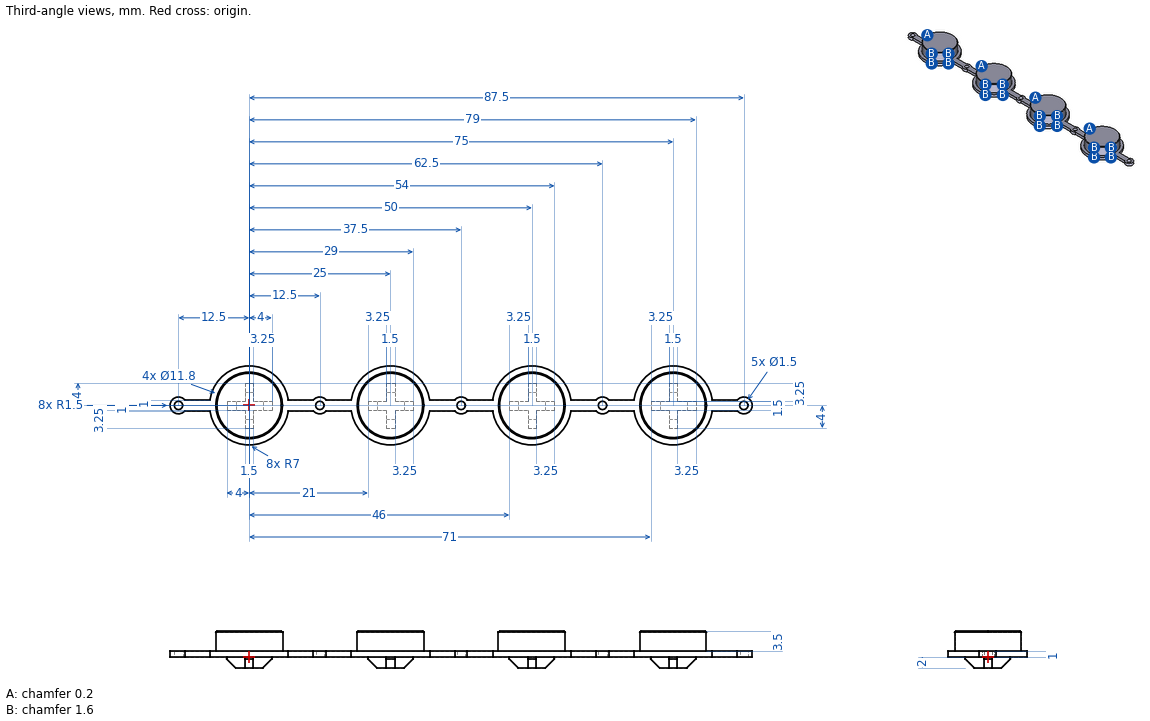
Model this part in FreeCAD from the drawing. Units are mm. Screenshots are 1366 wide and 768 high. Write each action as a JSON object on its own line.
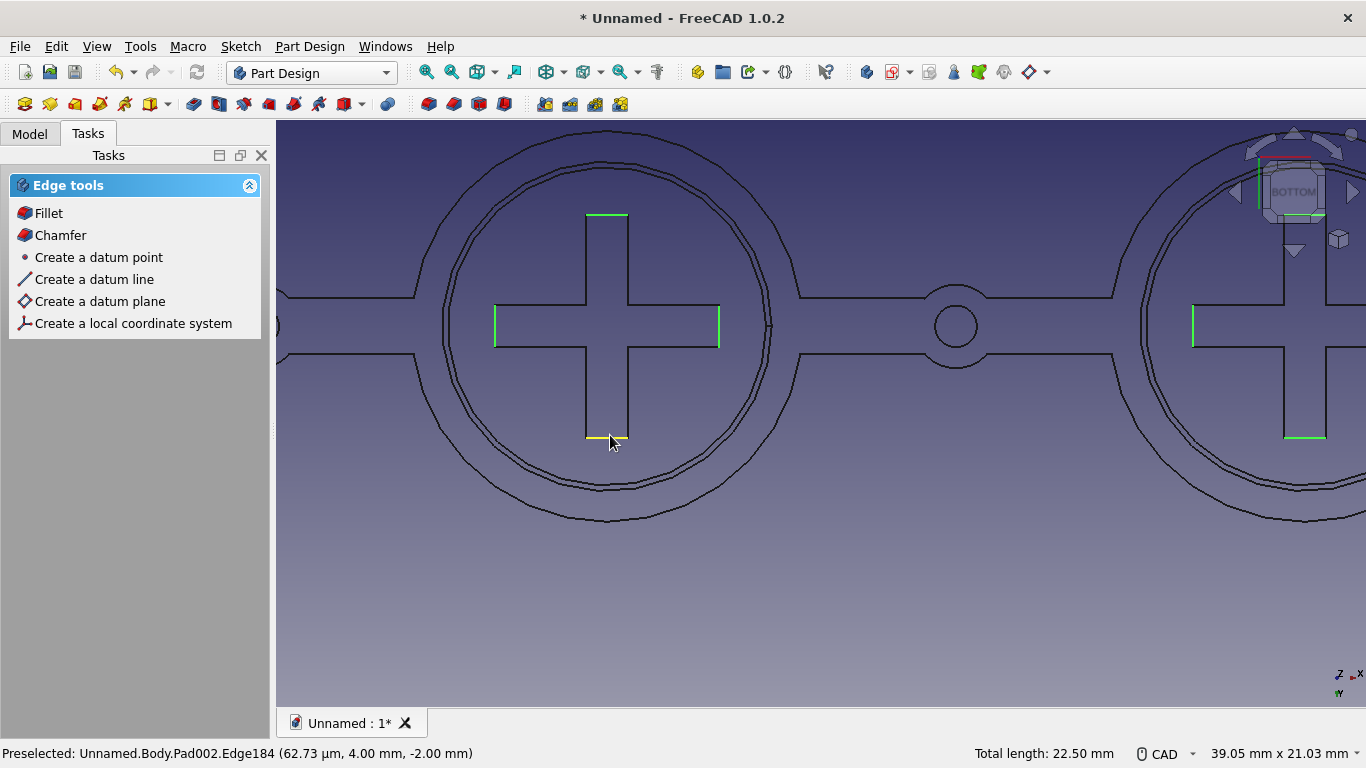
{"action": "left_click", "coordinate": [607, 437], "text": "ctrl"}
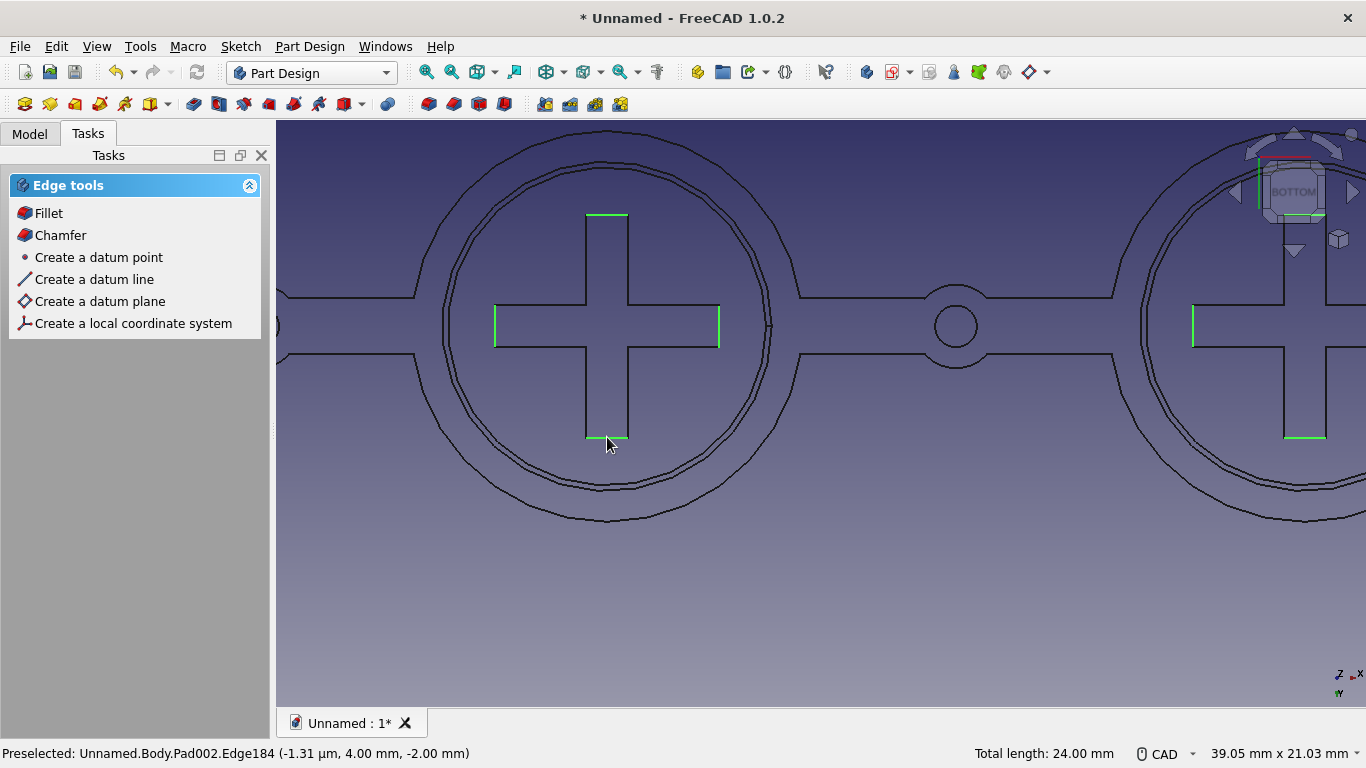
{"action": "key", "text": "v 1"}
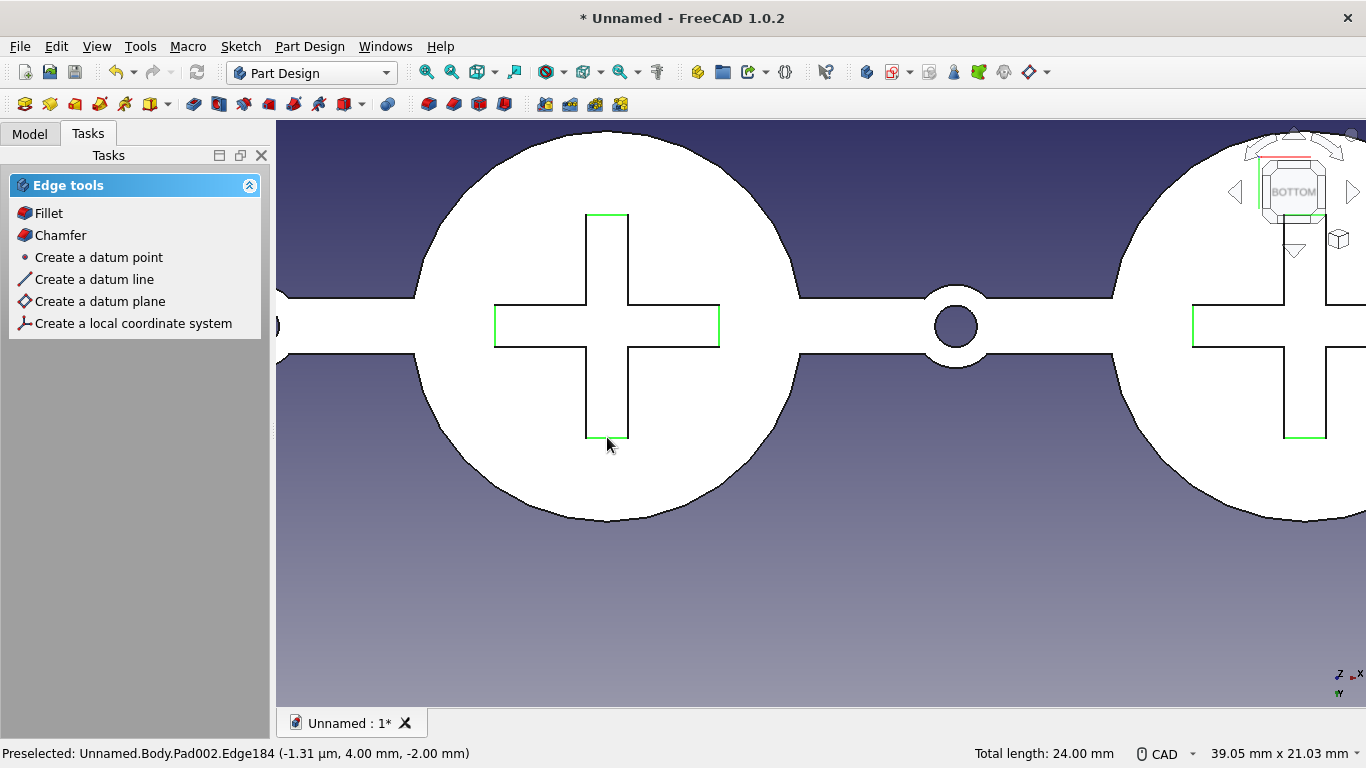
{"action": "left_click", "coordinate": [454, 104]}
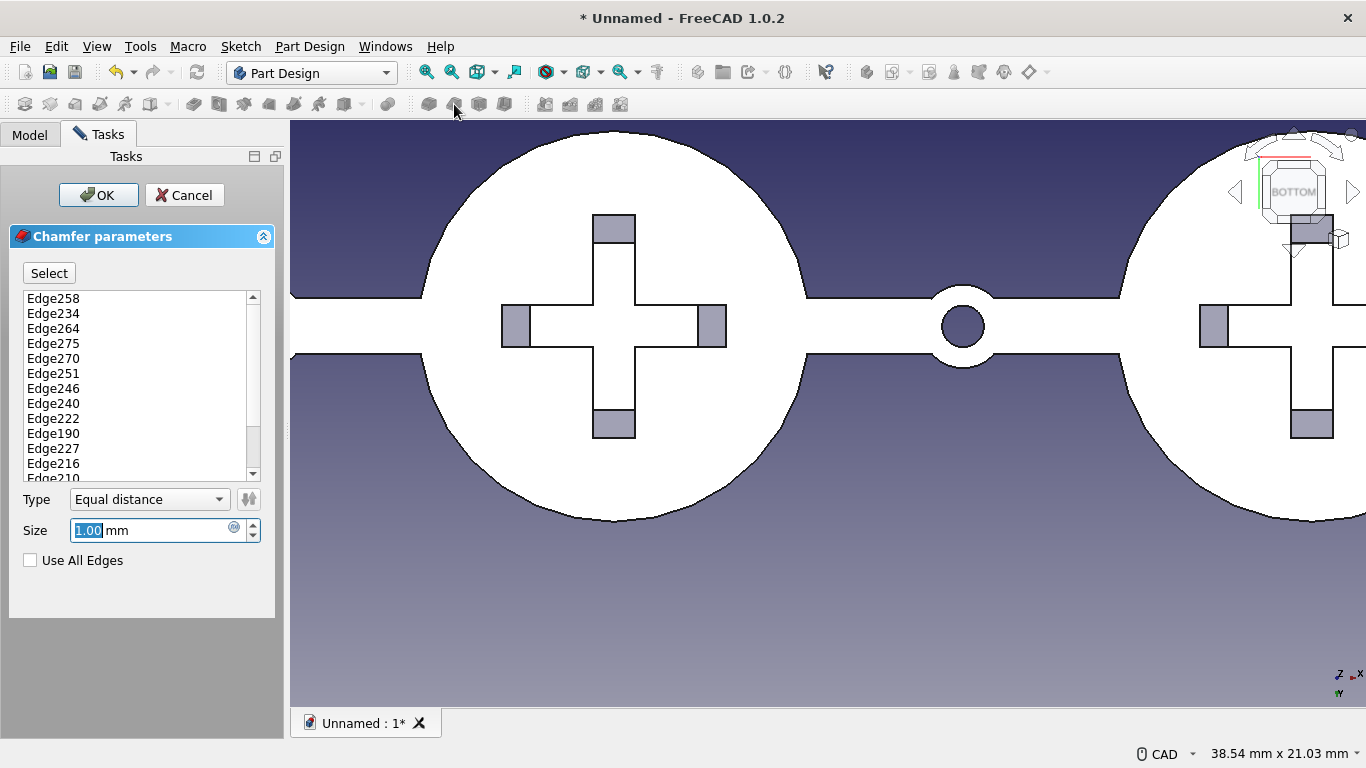
{"action": "type", "text": "1.6"}
{"action": "key", "text": "Tab"}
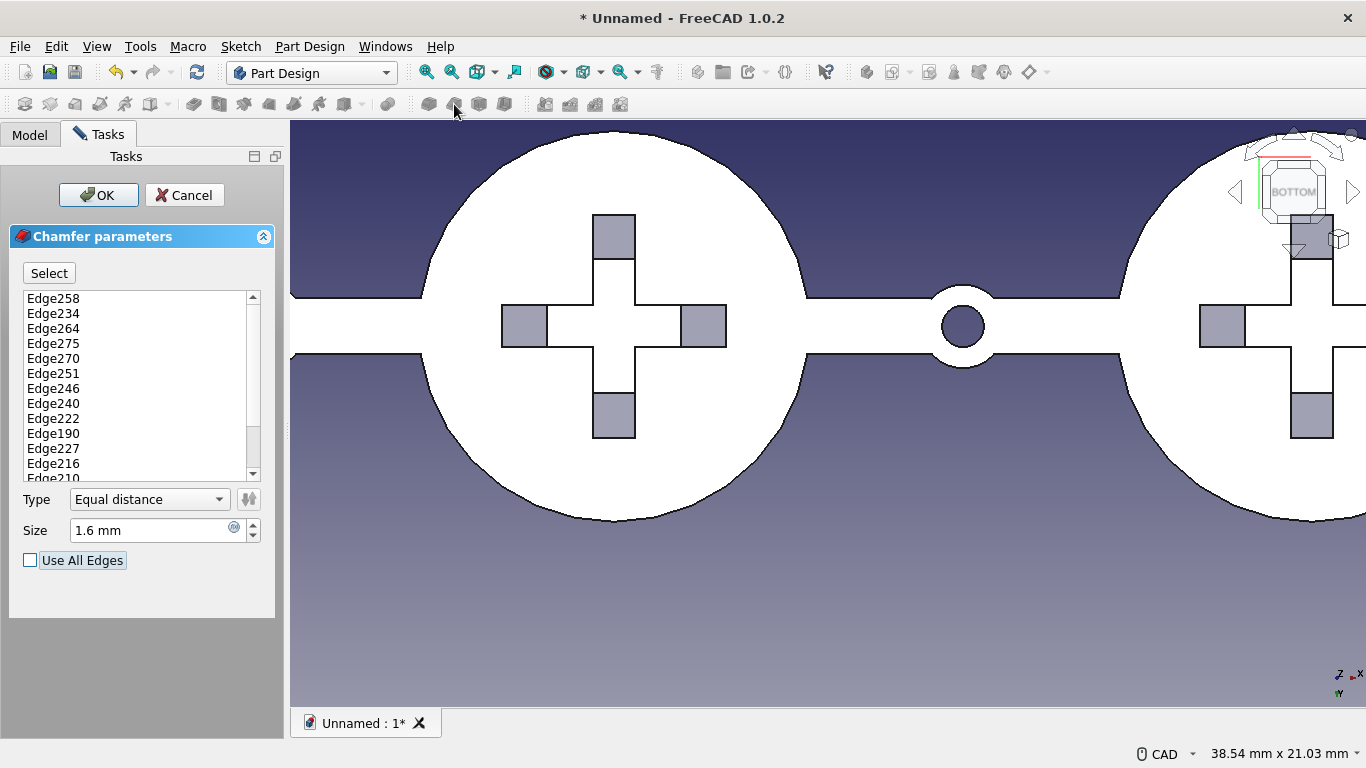
{"action": "left_click", "coordinate": [99, 195]}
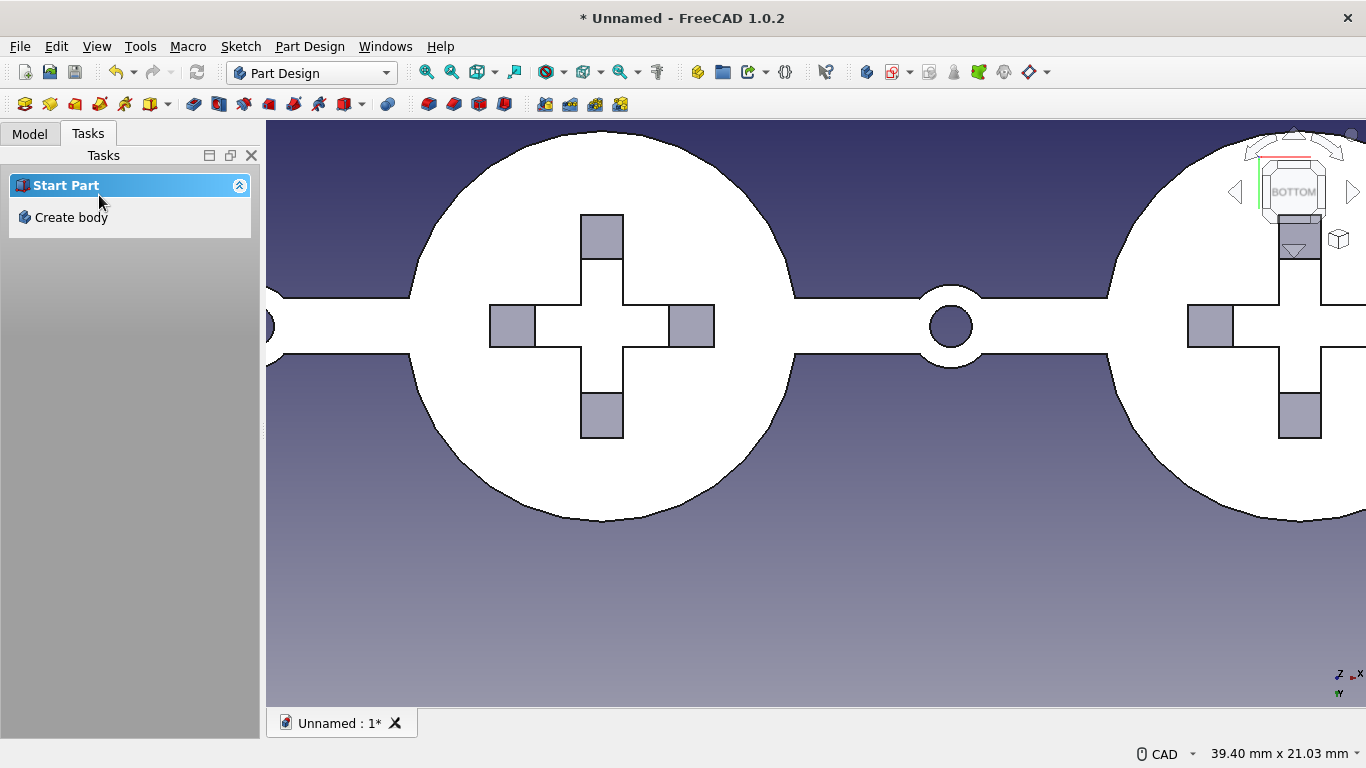
{"action": "key", "text": "0"}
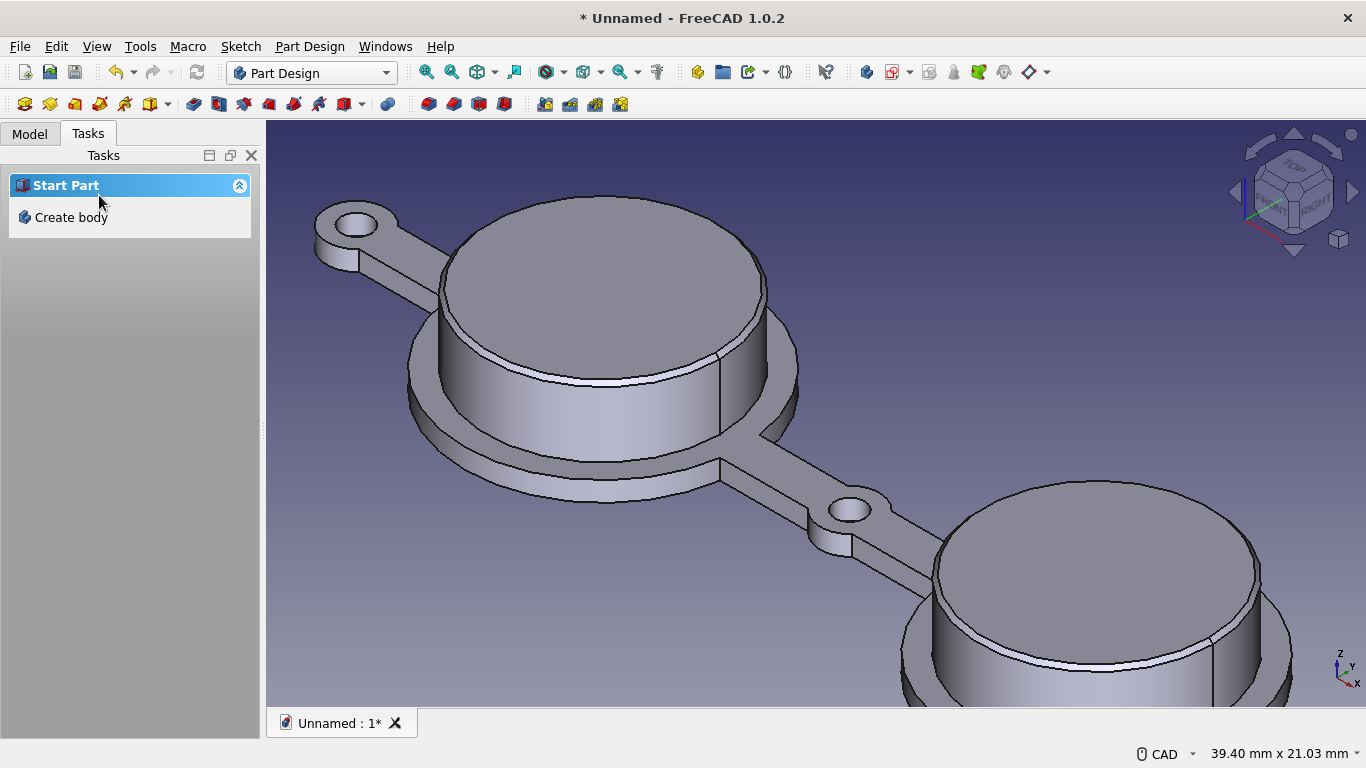
{"action": "key", "text": "v f"}